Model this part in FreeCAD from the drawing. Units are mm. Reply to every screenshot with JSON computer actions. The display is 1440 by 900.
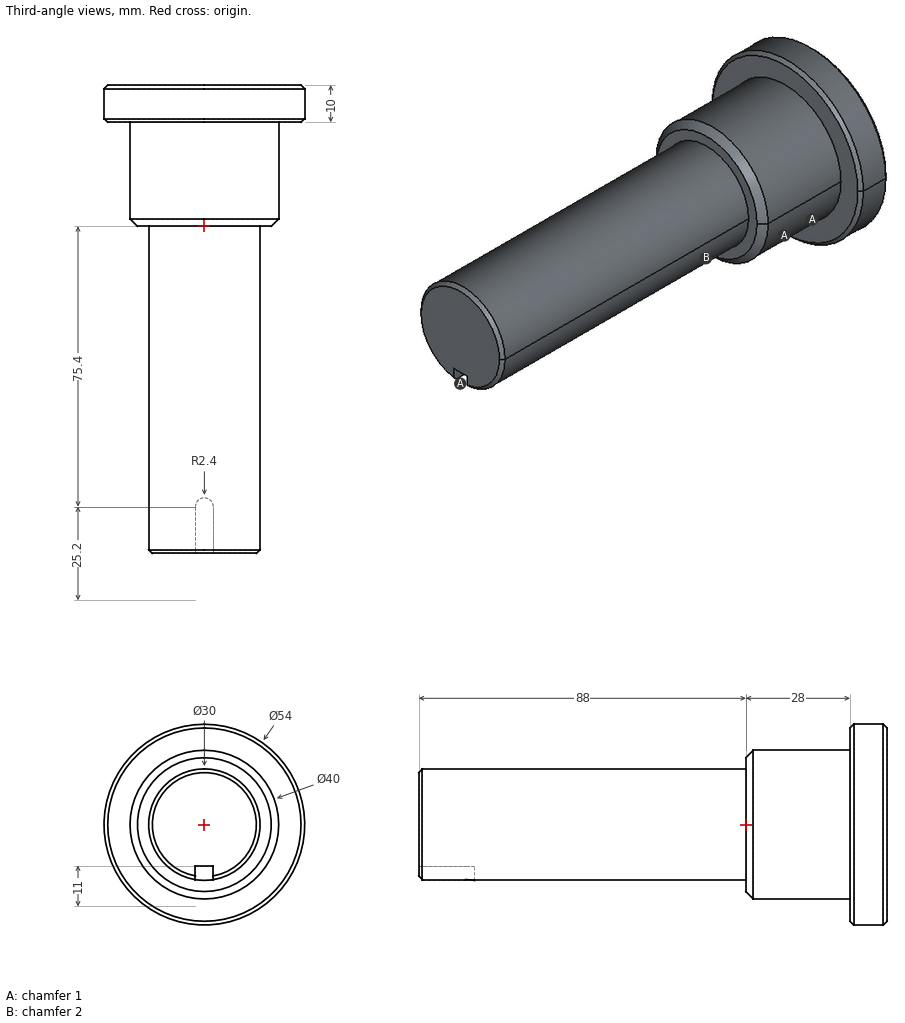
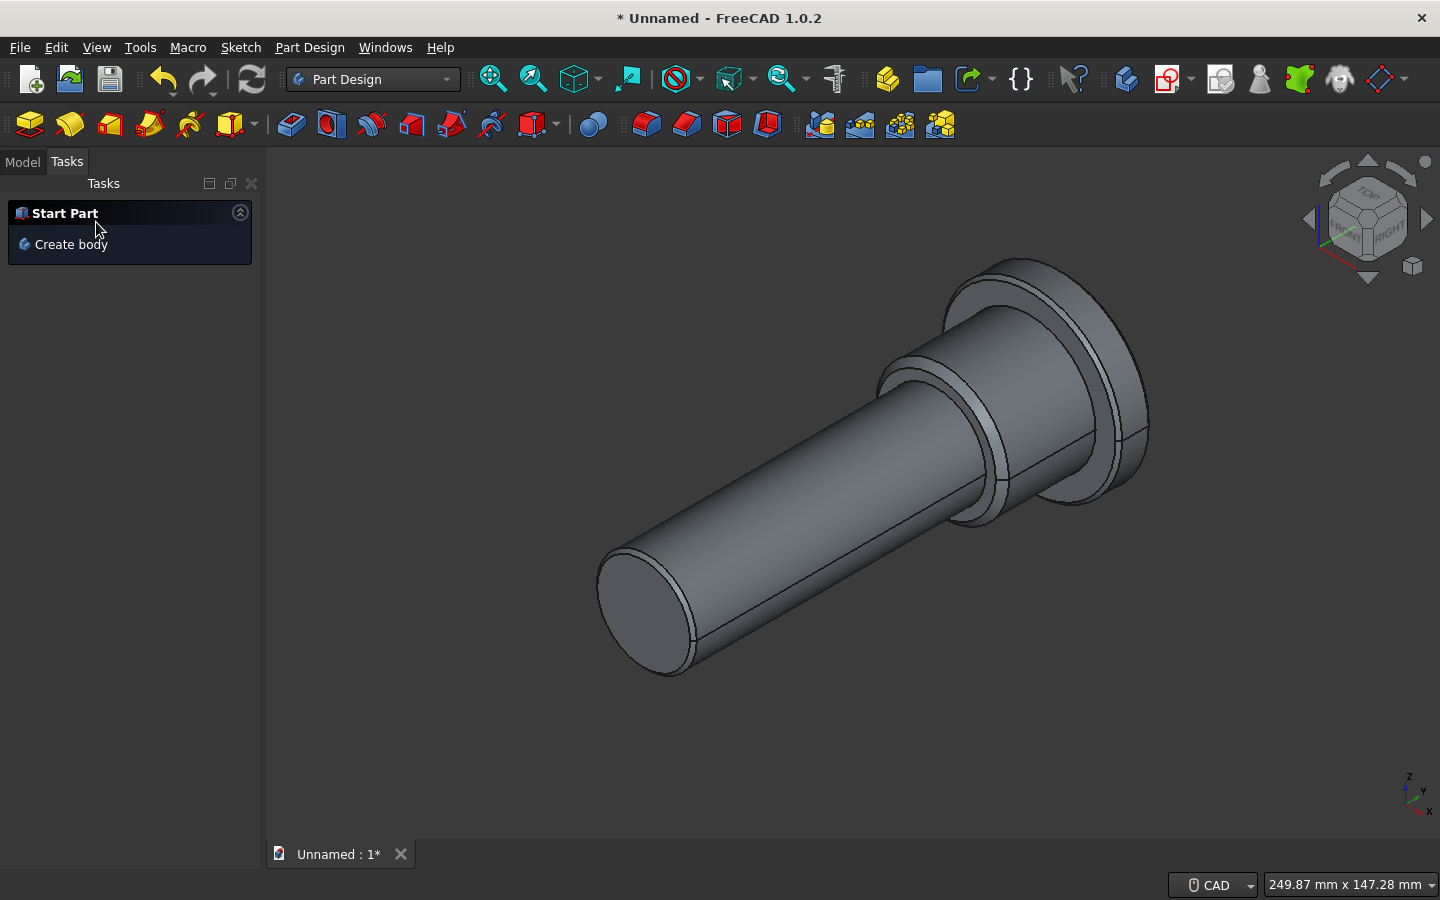
{"action": "left_click", "coordinate": [23, 161]}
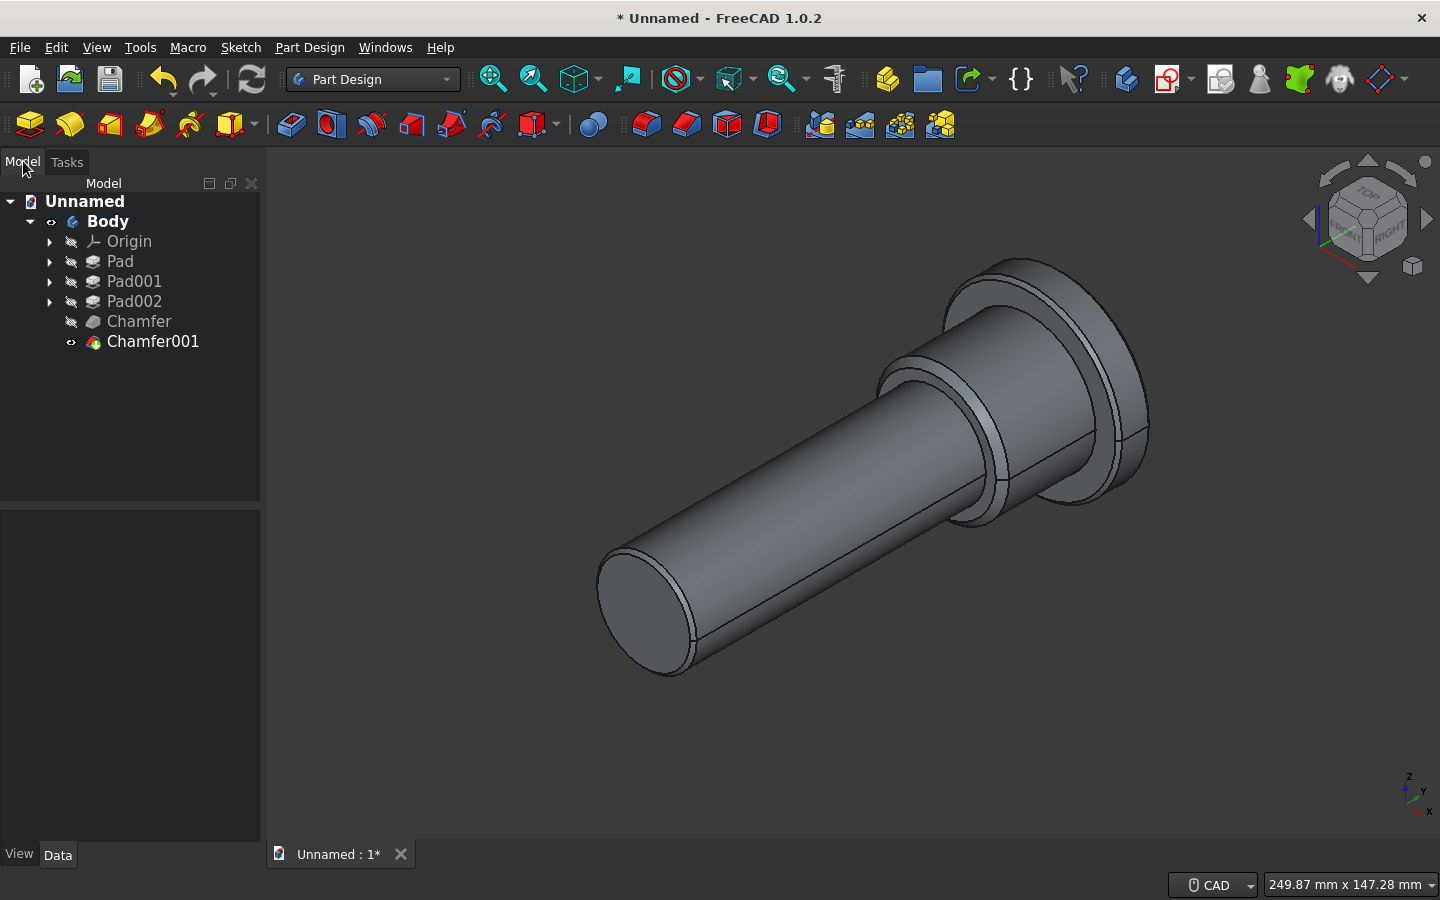
{"action": "left_click", "coordinate": [50, 242]}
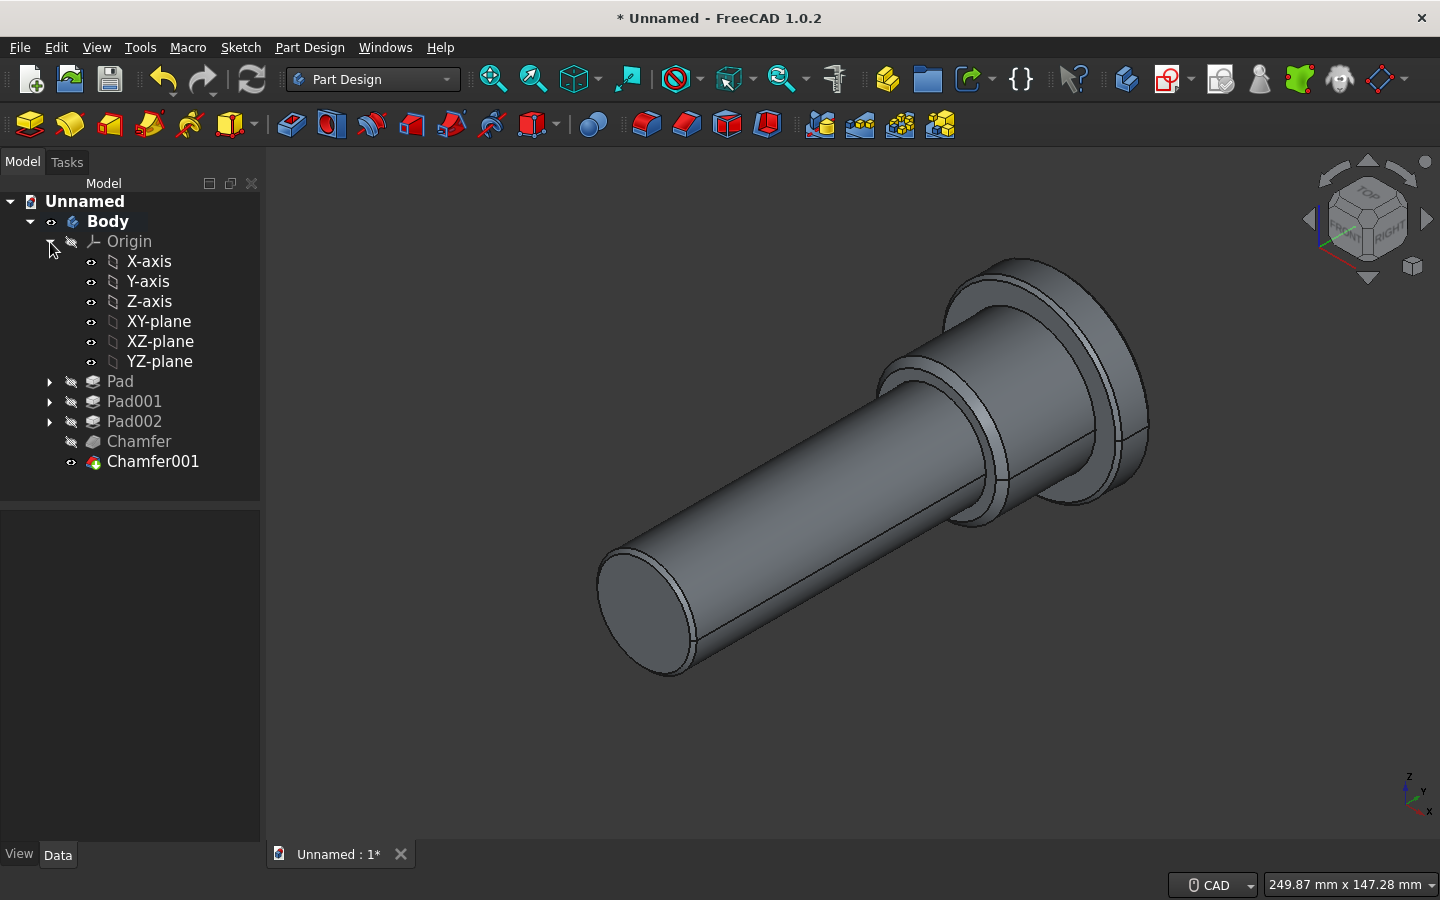
{"action": "left_click", "coordinate": [136, 322]}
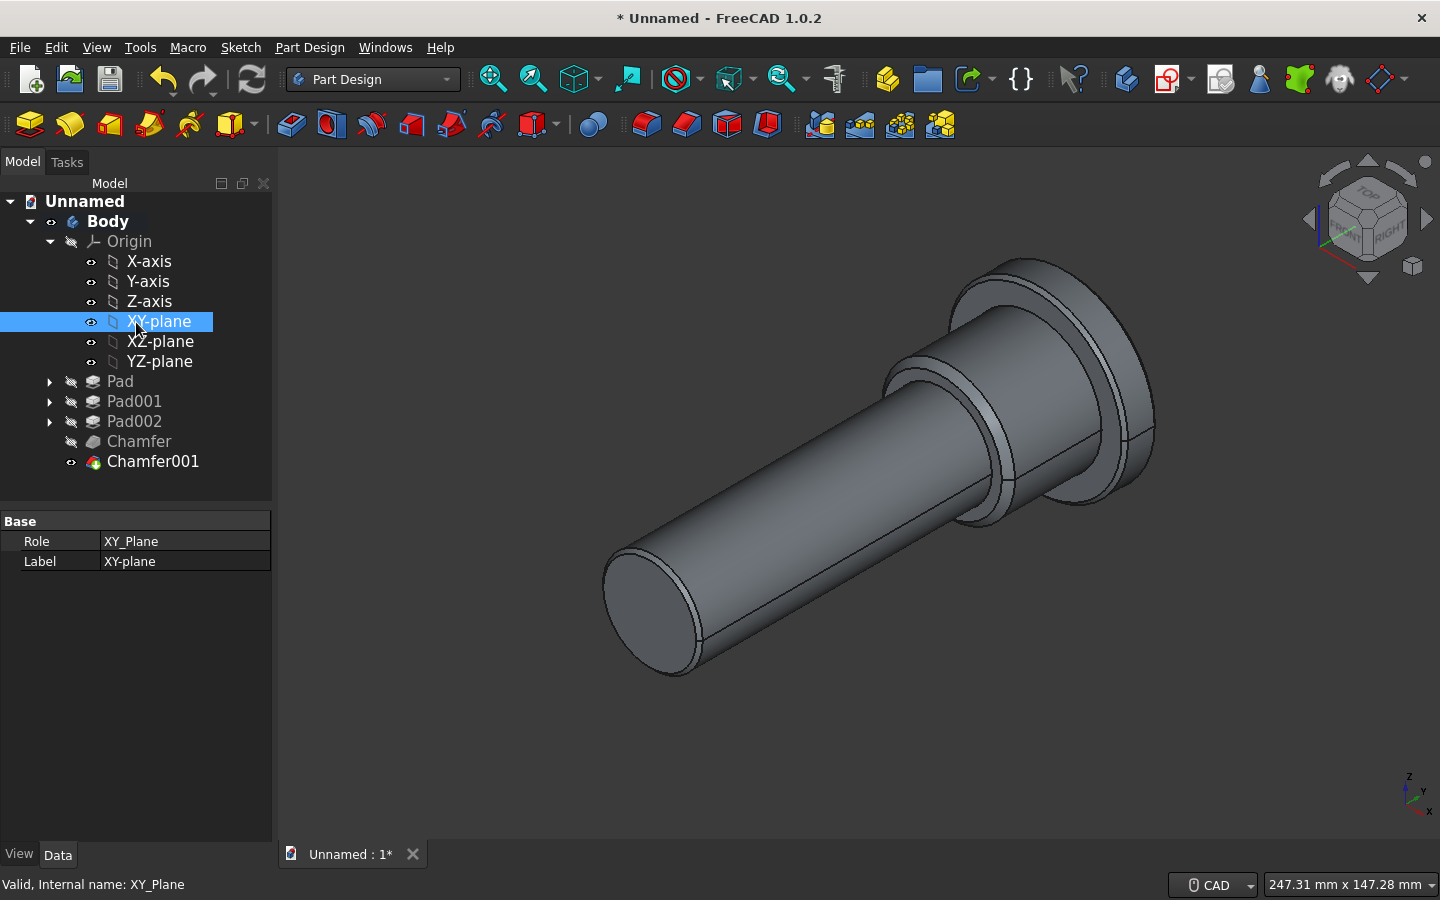
{"action": "left_click", "coordinate": [1380, 80]}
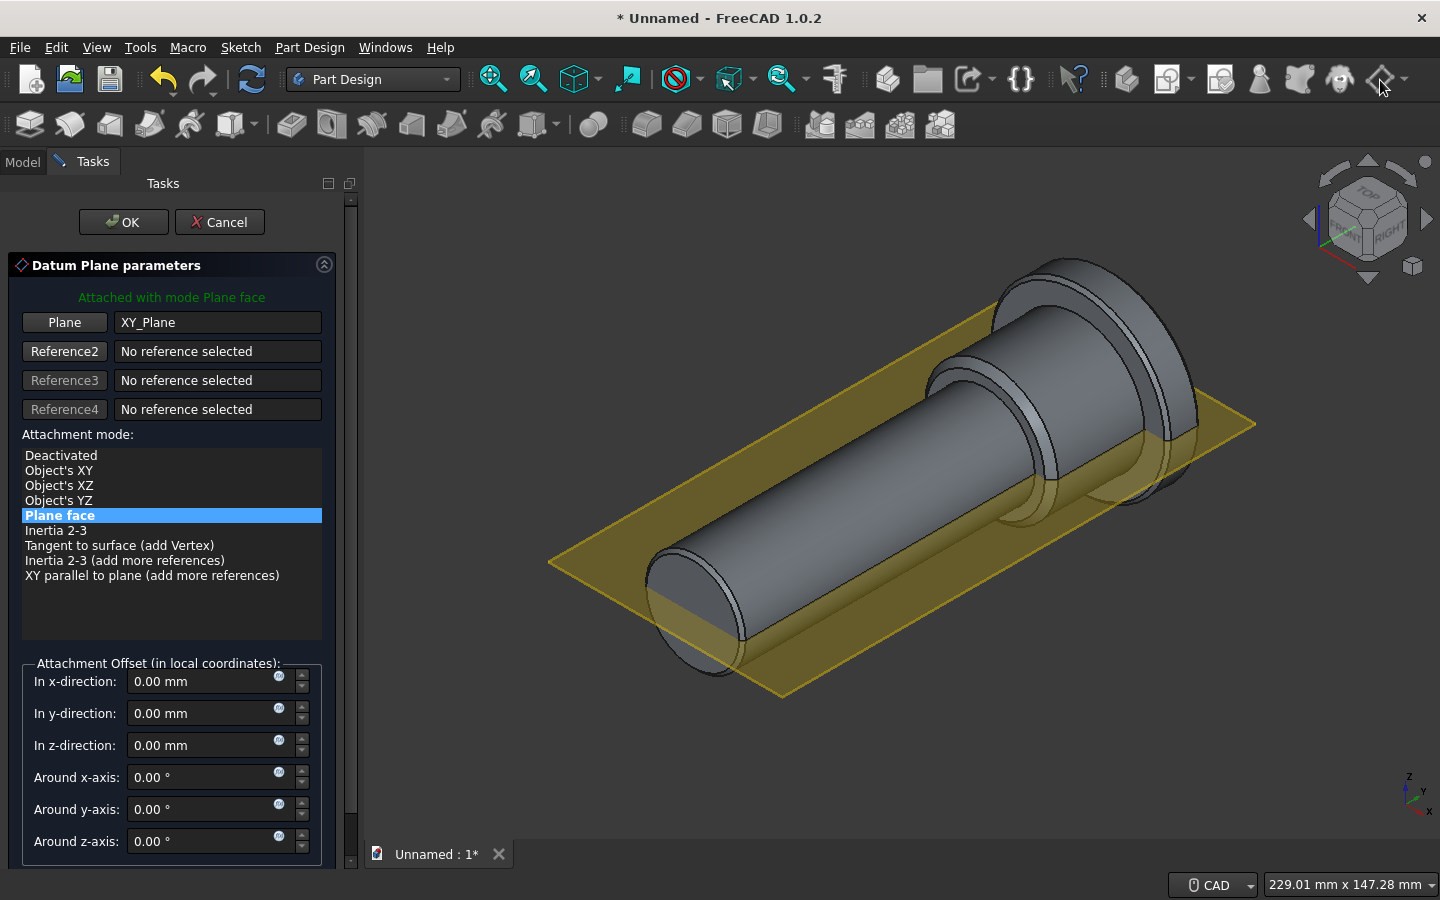
{"action": "triple_click", "coordinate": [210, 745]}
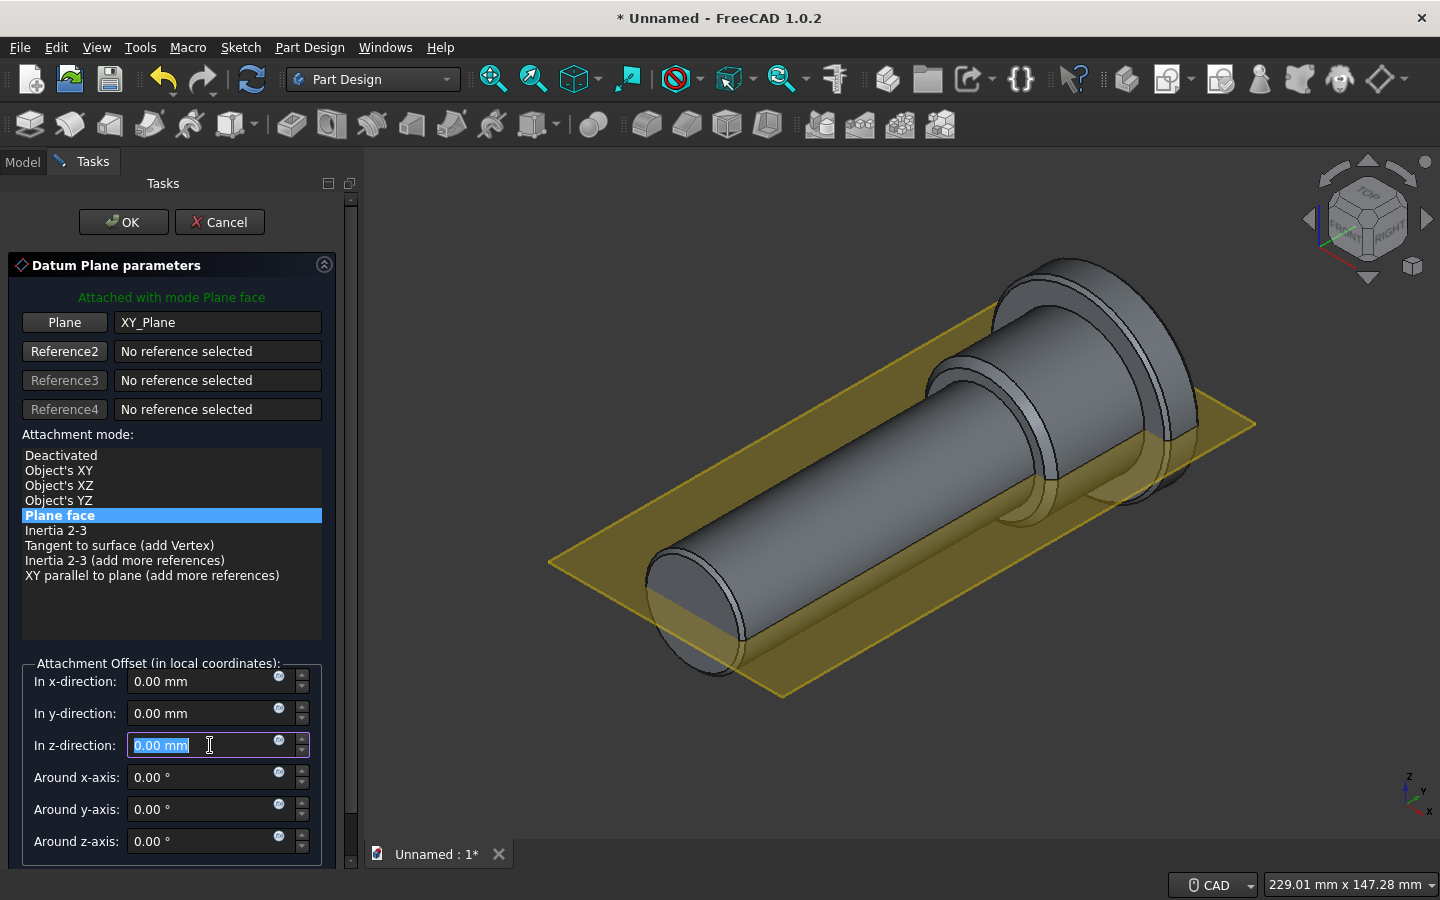
{"action": "type", "text": "-11"}
{"action": "key", "text": "Tab"}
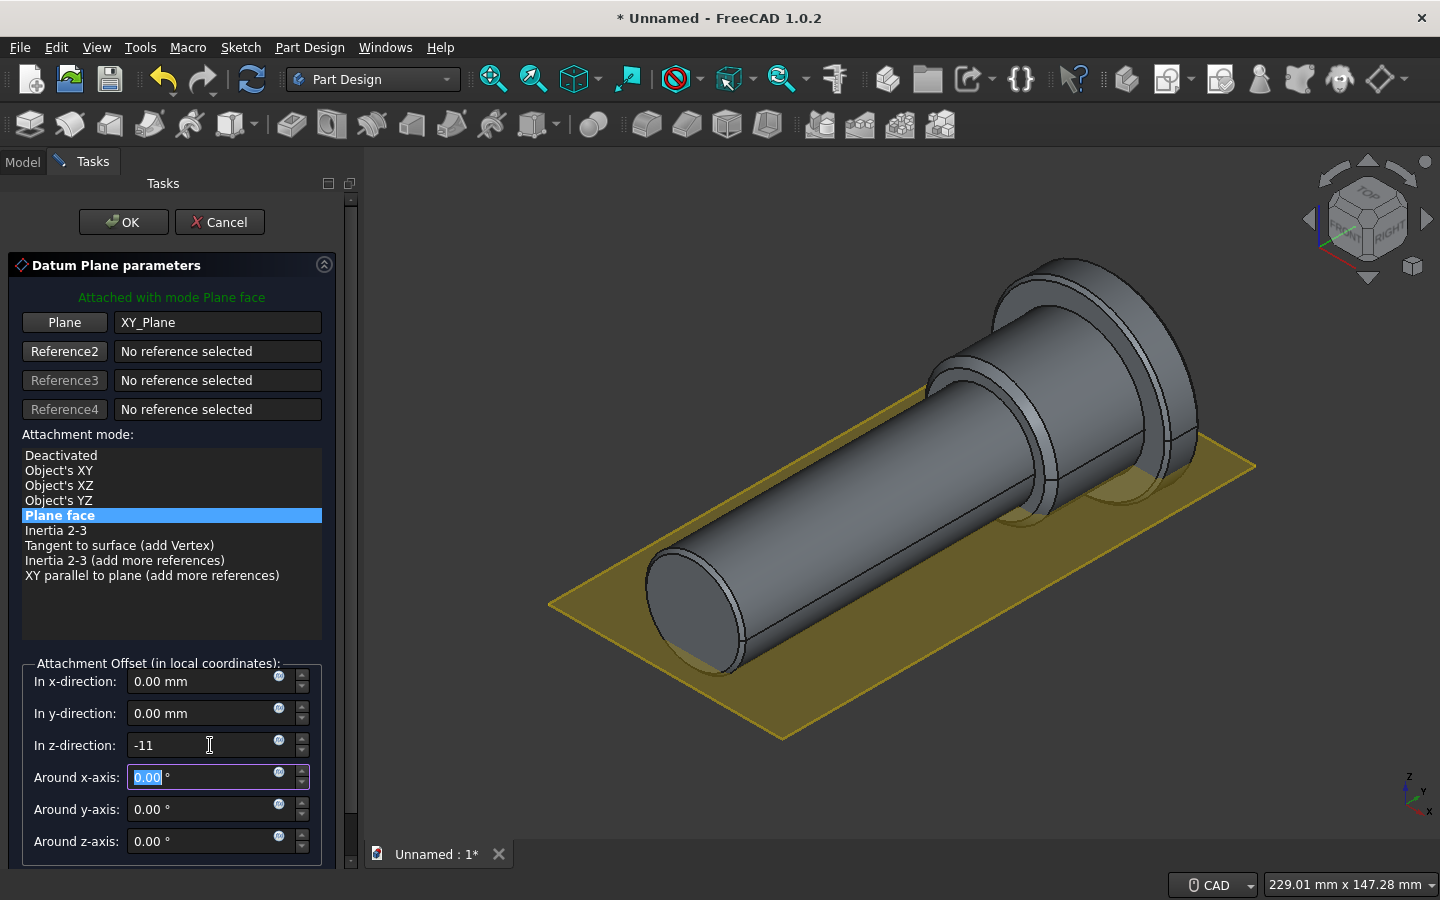
{"action": "left_click", "coordinate": [124, 222]}